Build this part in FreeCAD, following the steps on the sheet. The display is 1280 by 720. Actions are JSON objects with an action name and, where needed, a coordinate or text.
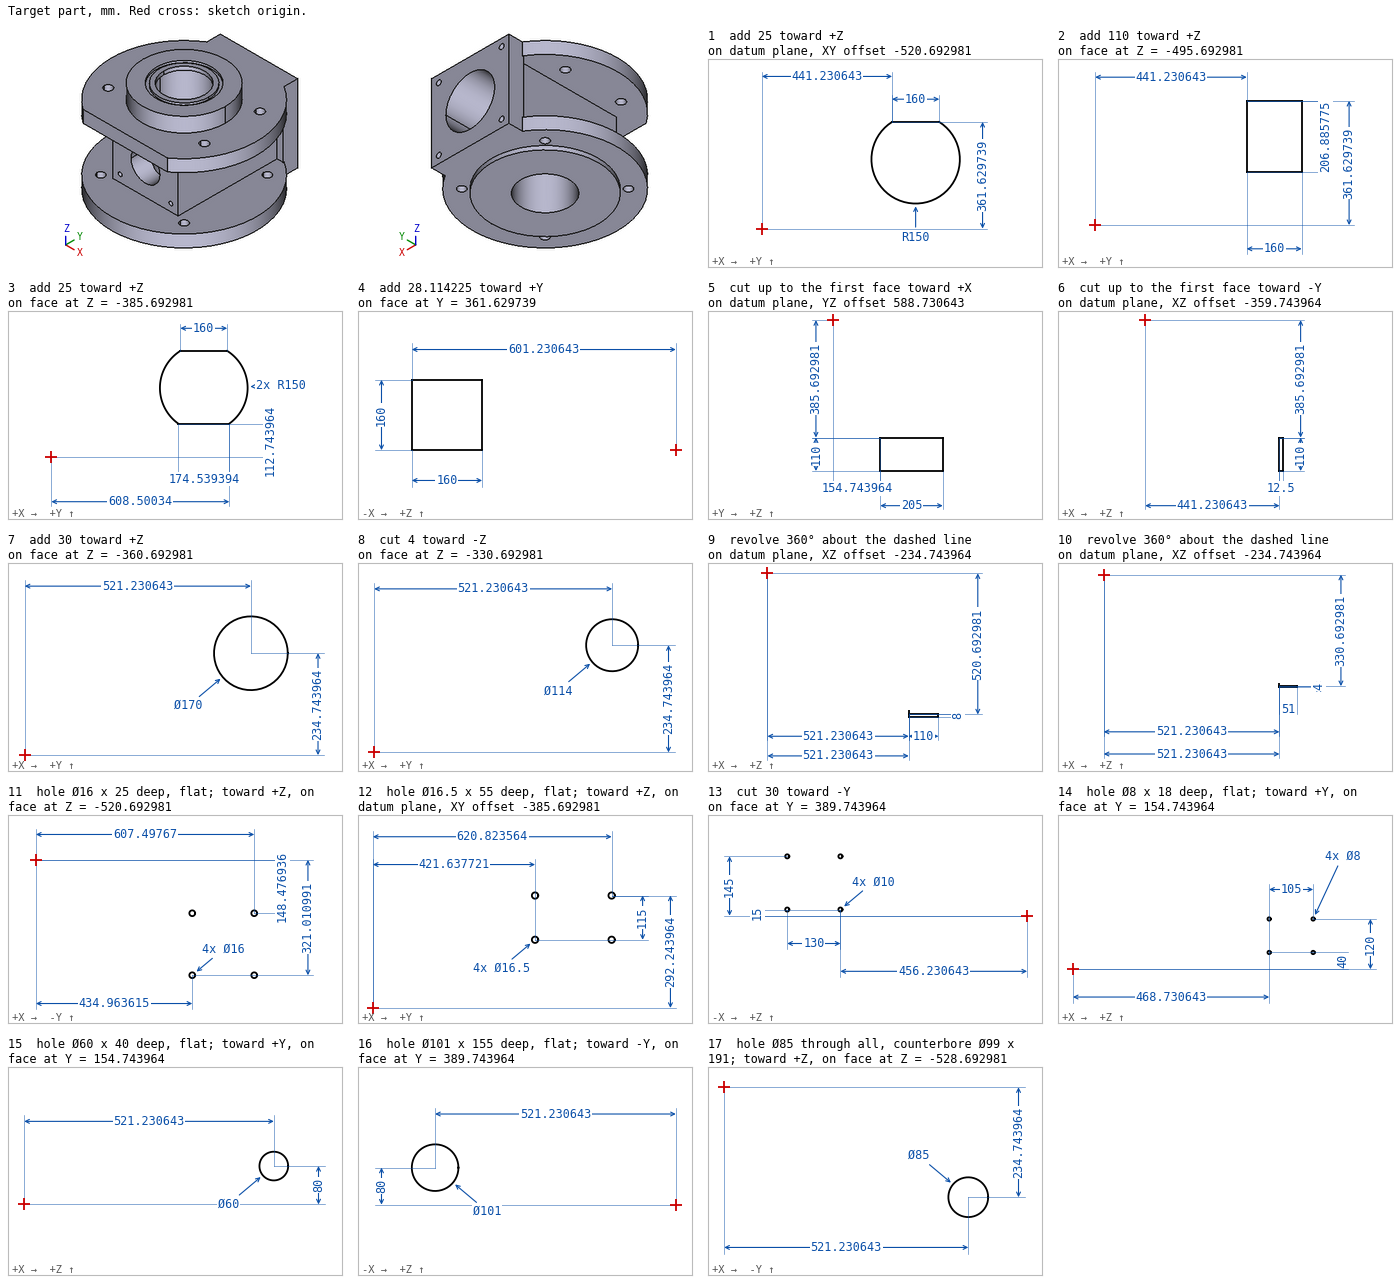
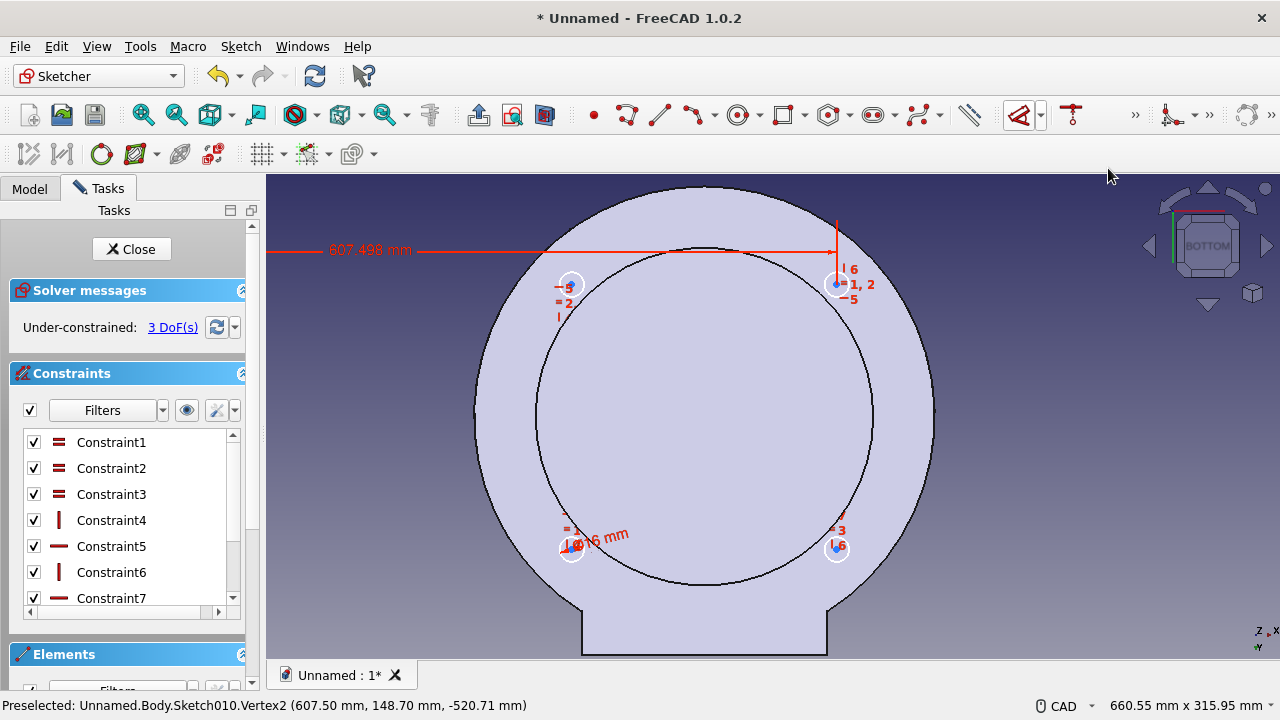
{"action": "left_click", "coordinate": [572, 550]}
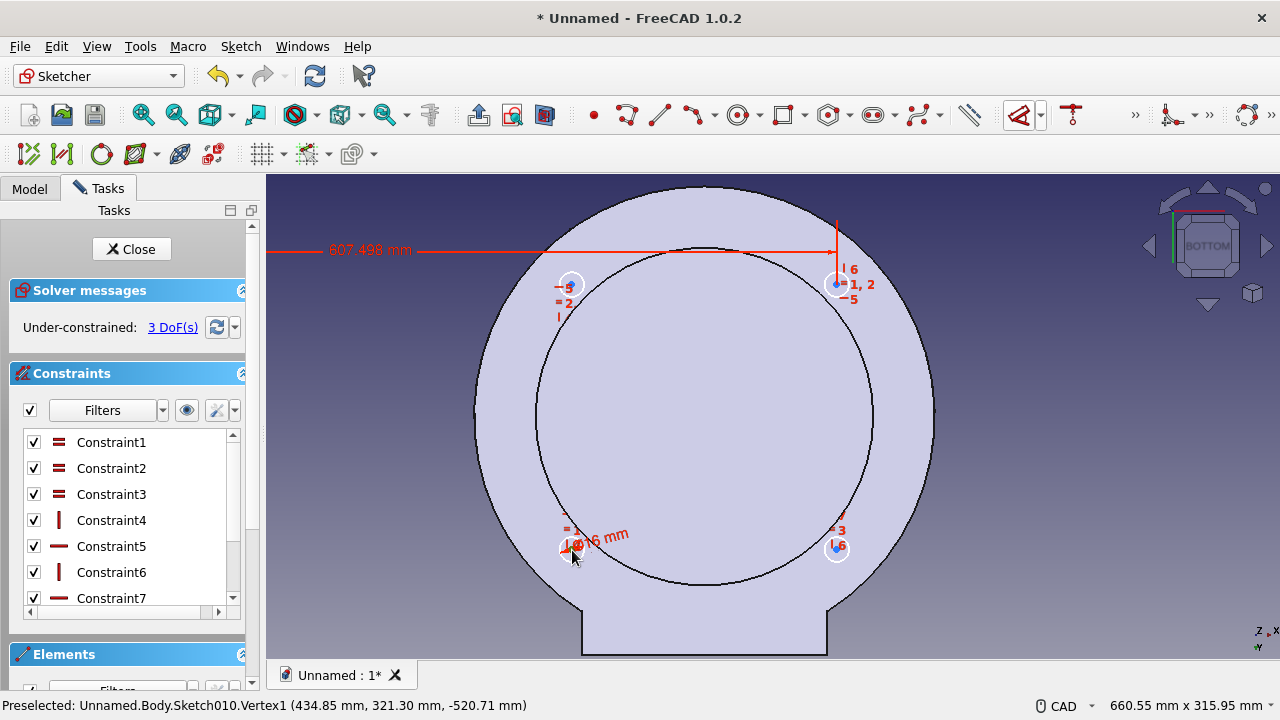
{"action": "left_click", "coordinate": [1040, 116]}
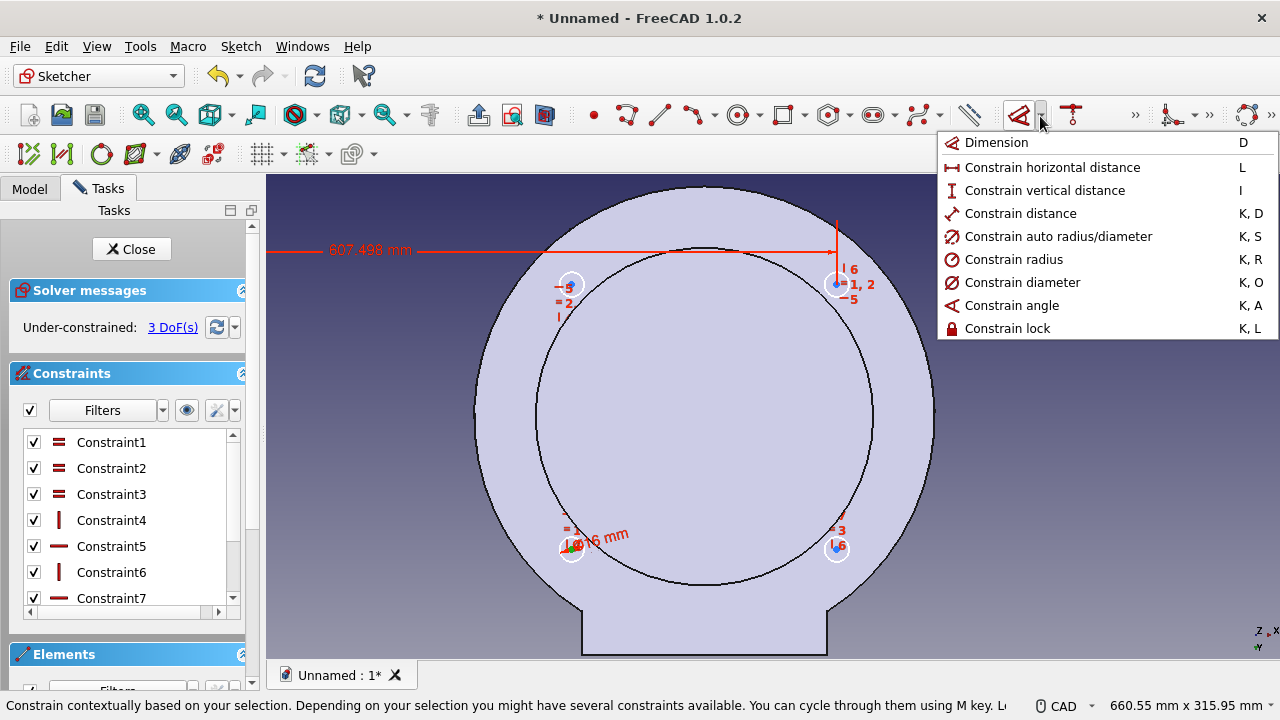
{"action": "left_click", "coordinate": [1108, 168]}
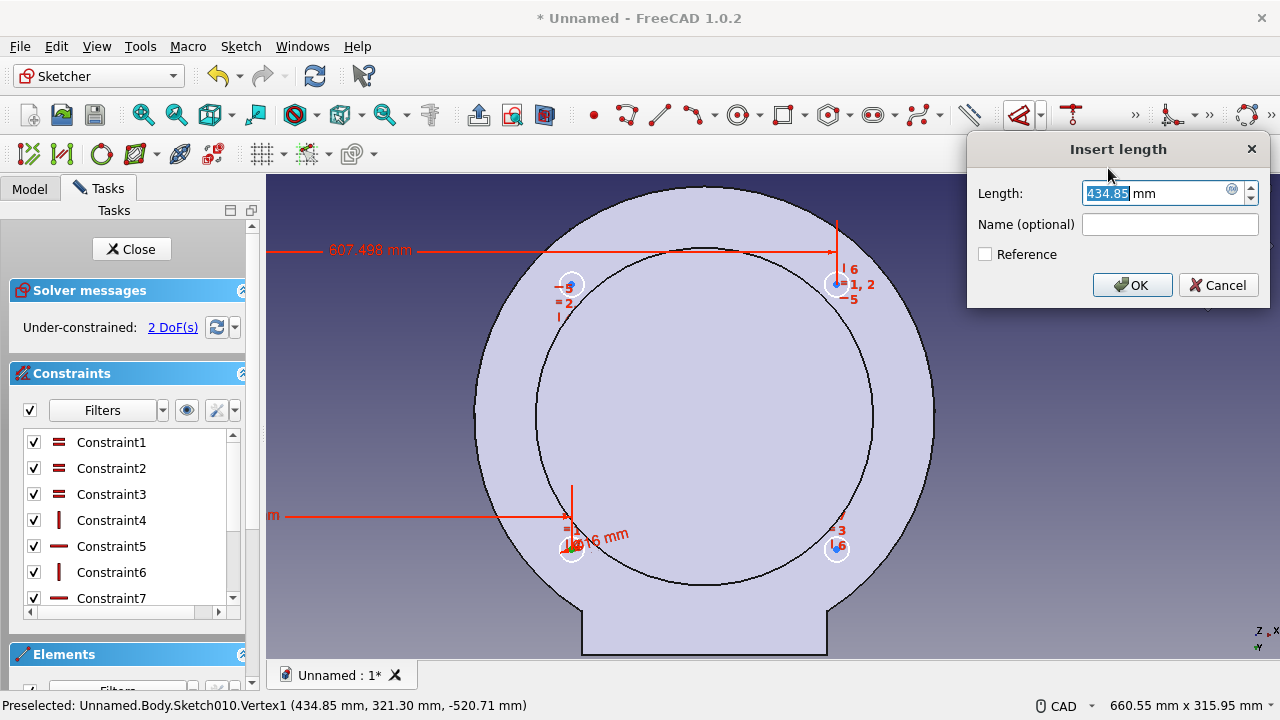
{"action": "type", "text": "434.963615"}
{"action": "key", "text": "Return"}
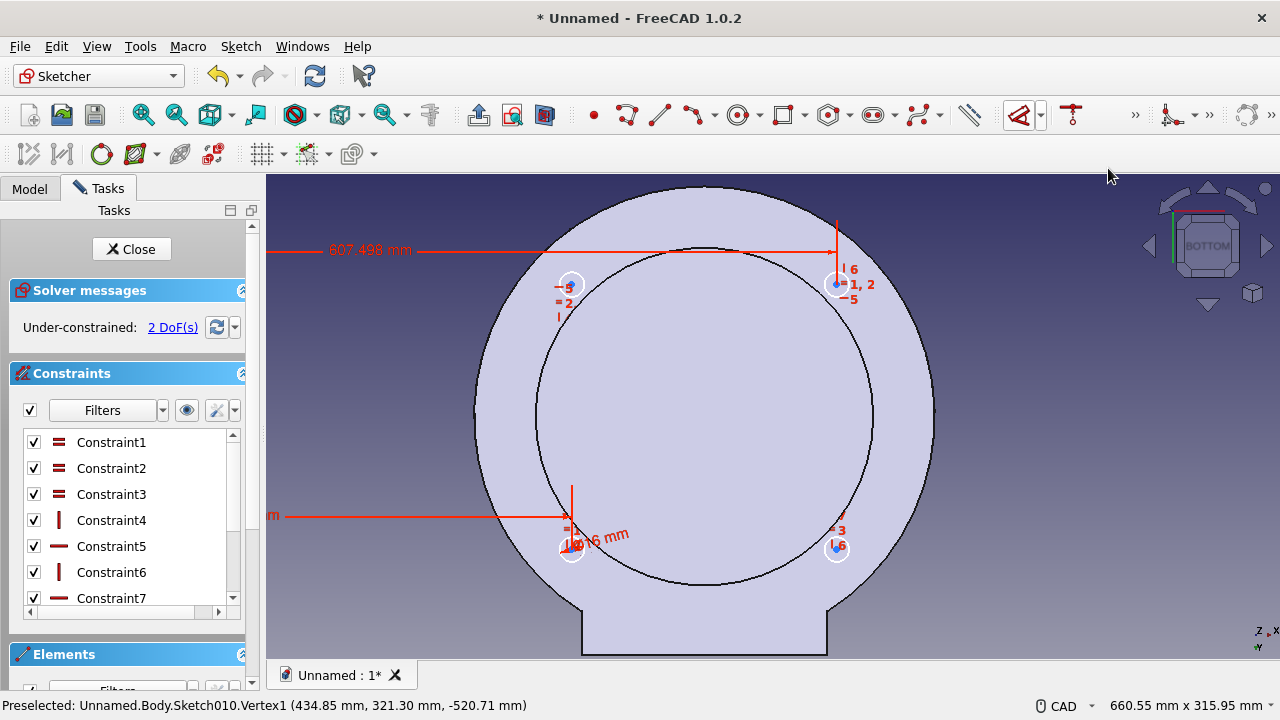
{"action": "left_click", "coordinate": [572, 550]}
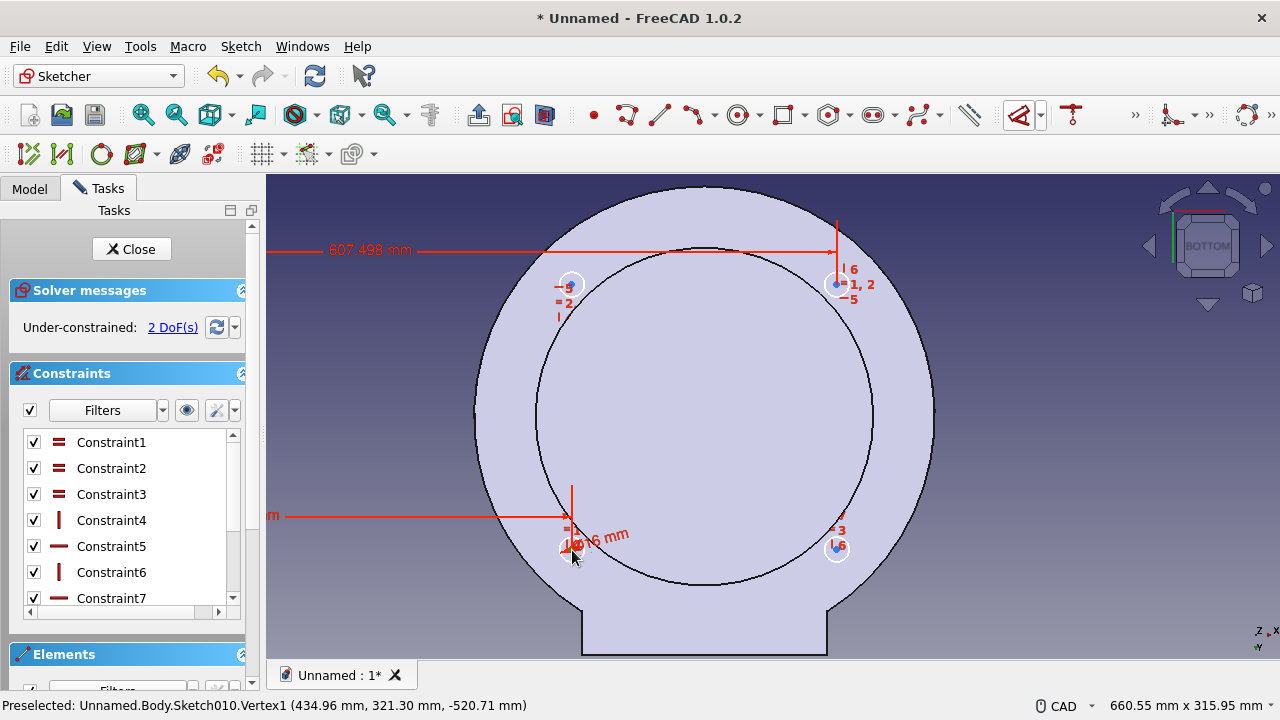
{"action": "left_click", "coordinate": [1040, 116]}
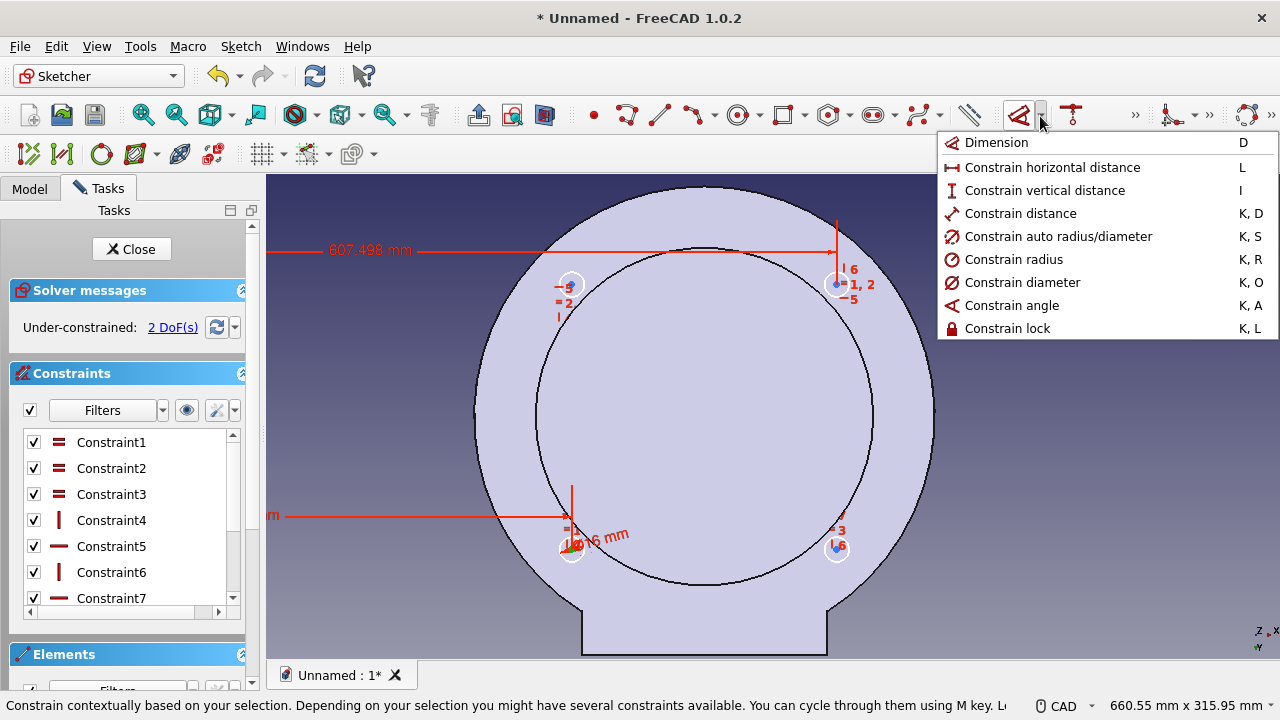
{"action": "left_click", "coordinate": [1108, 190]}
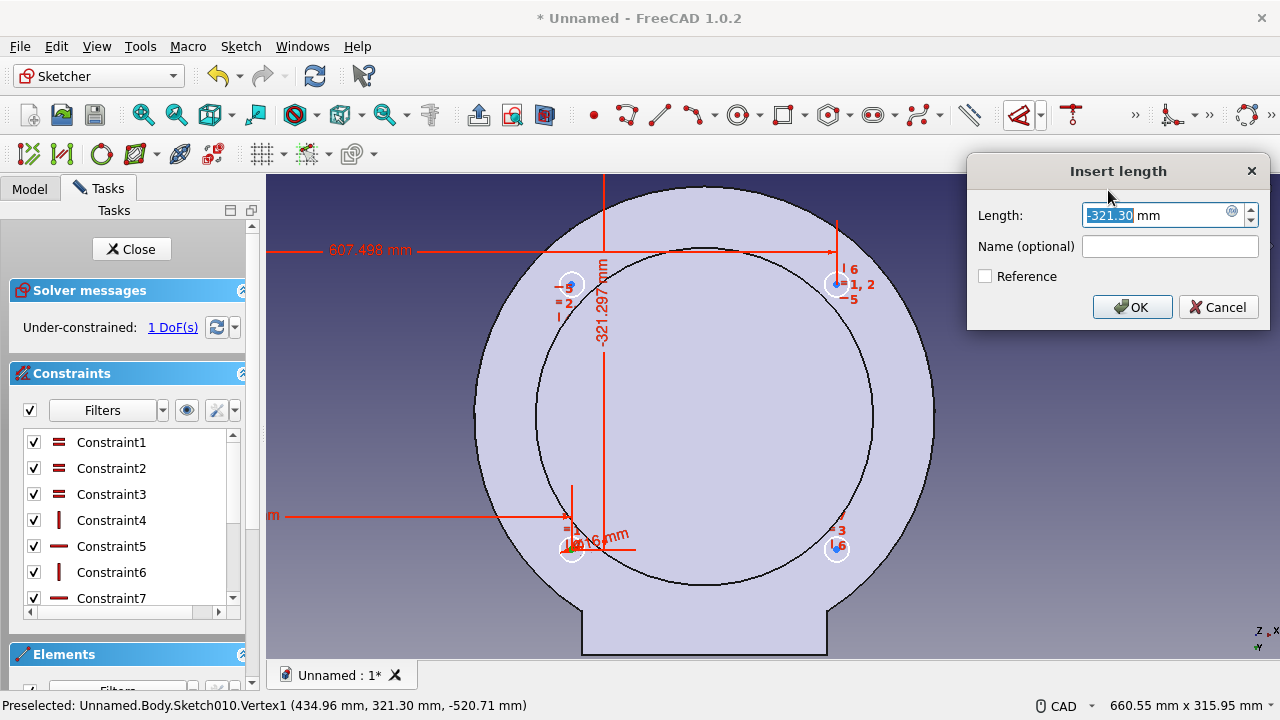
{"action": "type", "text": "-321.010991"}
{"action": "key", "text": "Return"}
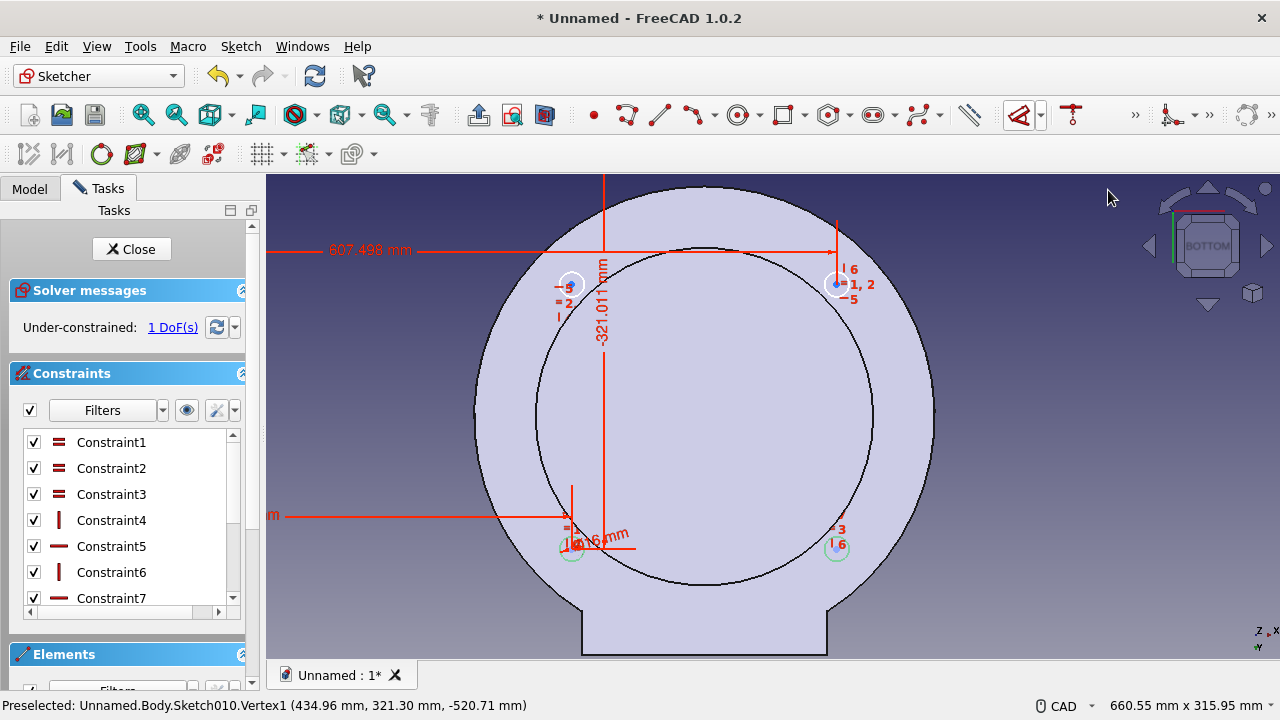
{"action": "left_click", "coordinate": [837, 285]}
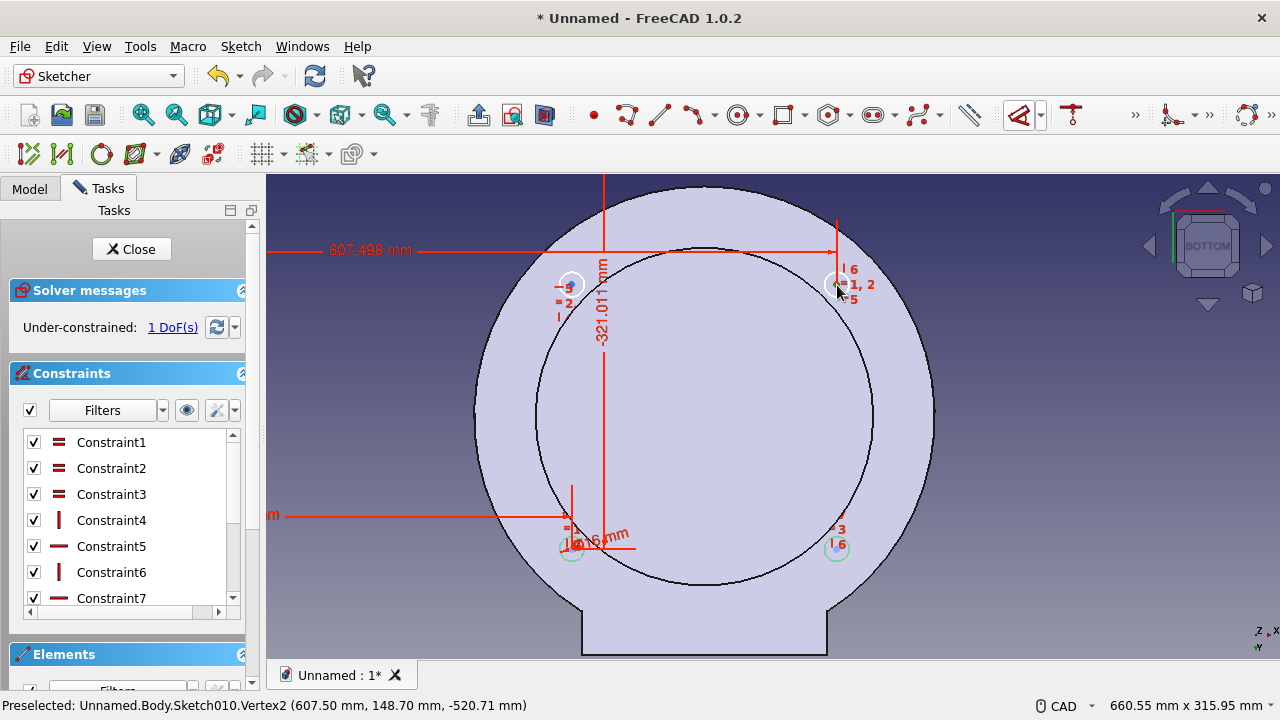
{"action": "left_click", "coordinate": [1040, 116]}